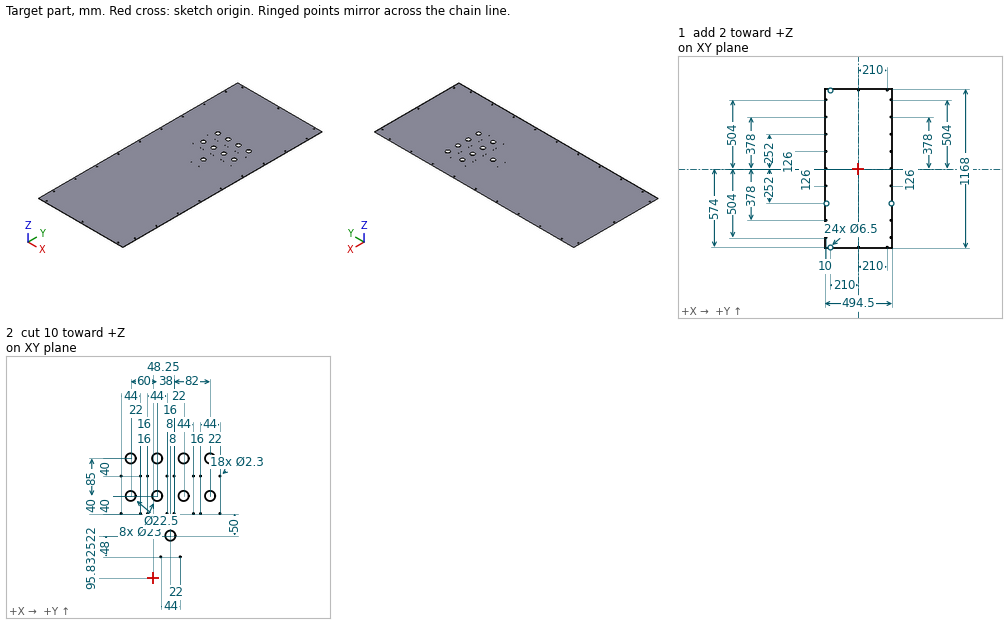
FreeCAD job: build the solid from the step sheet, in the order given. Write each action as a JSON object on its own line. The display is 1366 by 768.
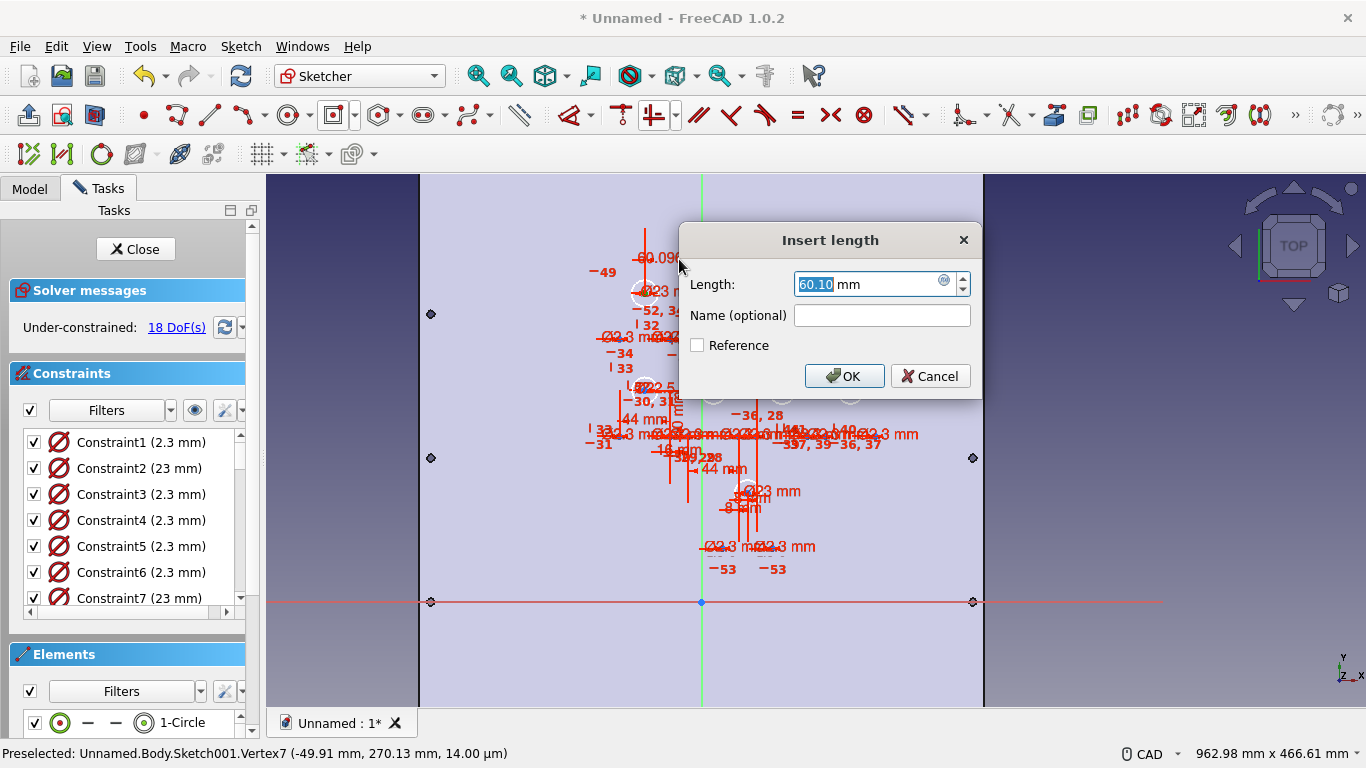
{"action": "type", "text": "60"}
{"action": "key", "text": "Return"}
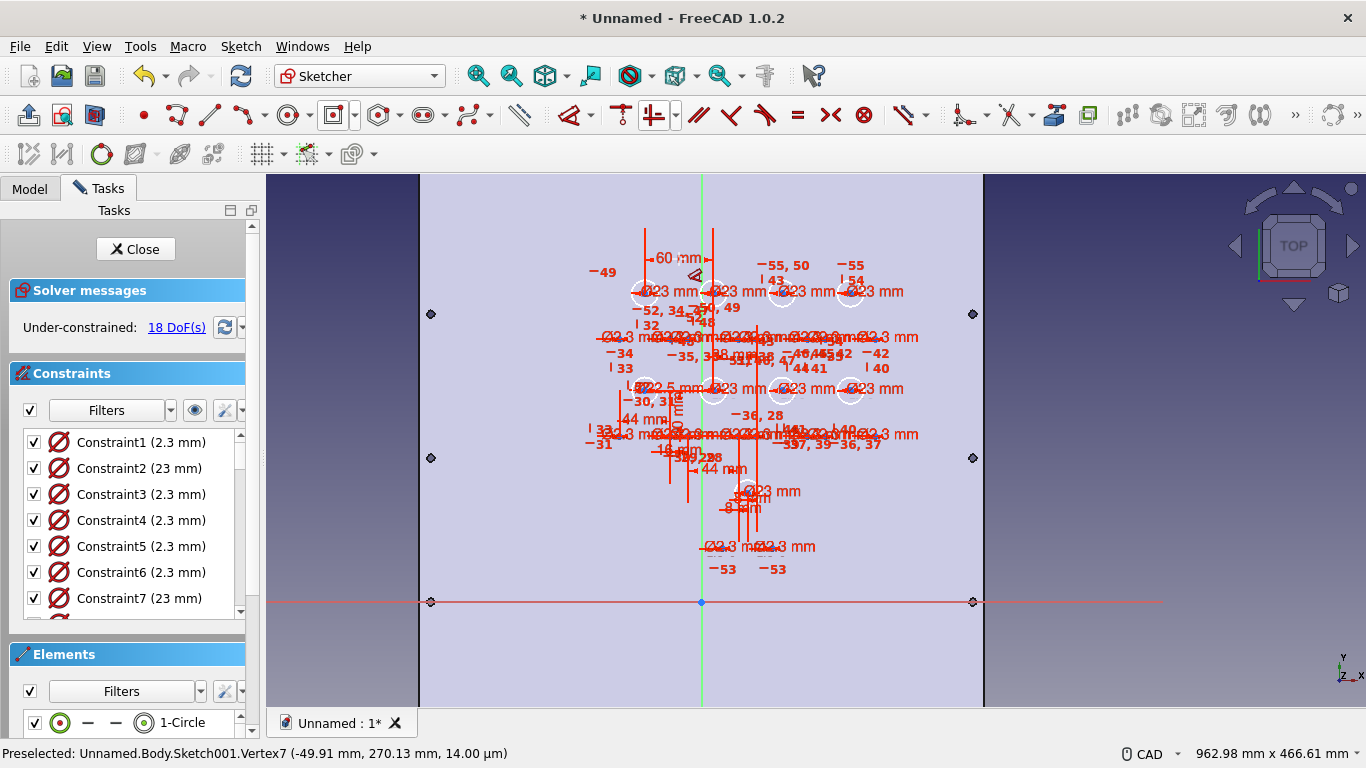
{"action": "left_click", "coordinate": [713, 391]}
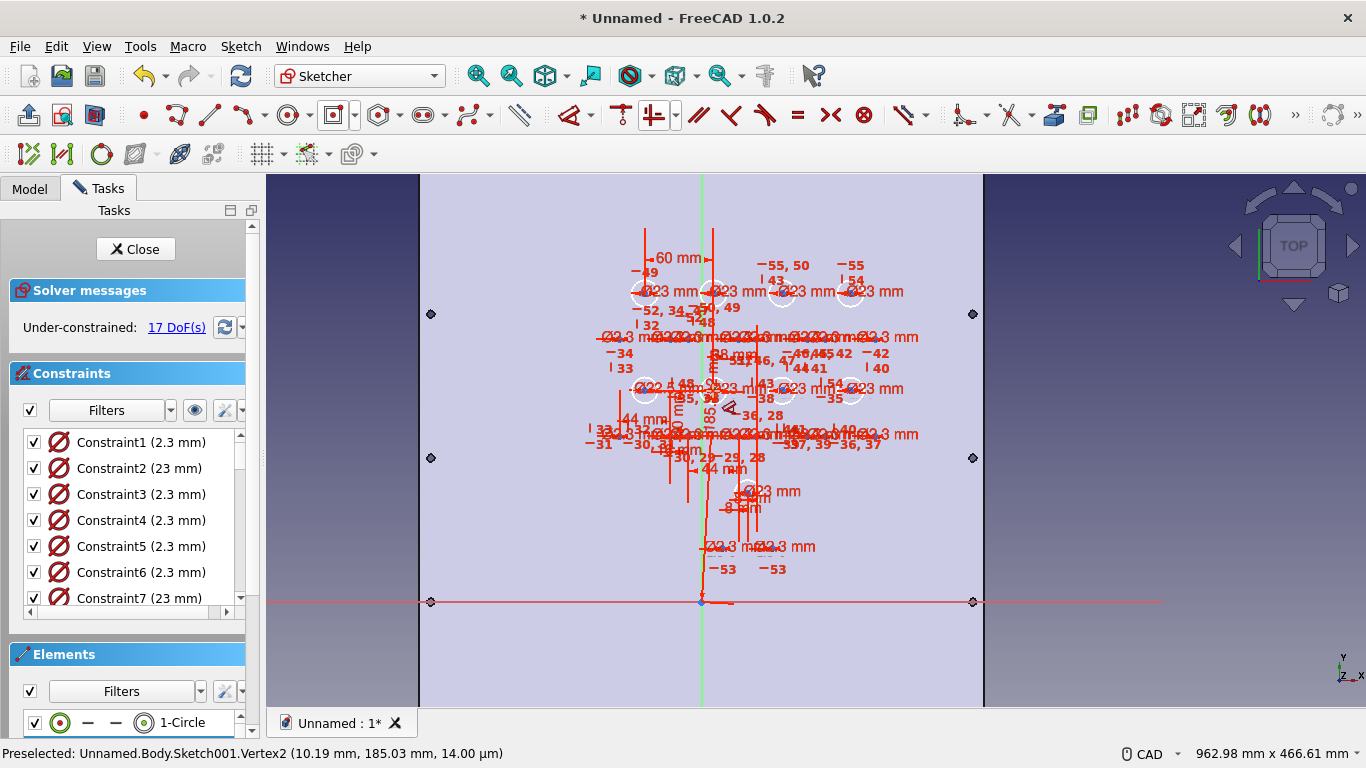
{"action": "left_click", "coordinate": [645, 293]}
{"action": "left_click", "coordinate": [611, 320]}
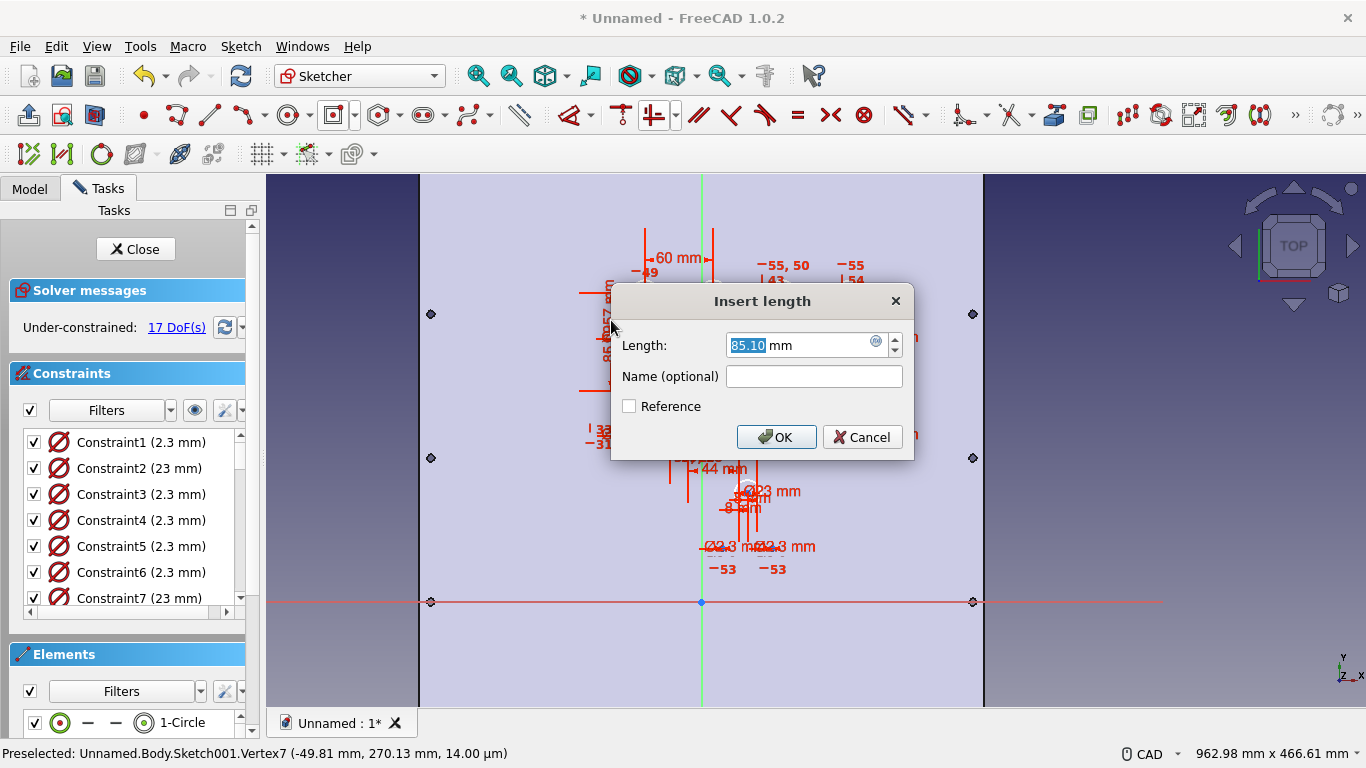
{"action": "type", "text": "85"}
{"action": "key", "text": "Return"}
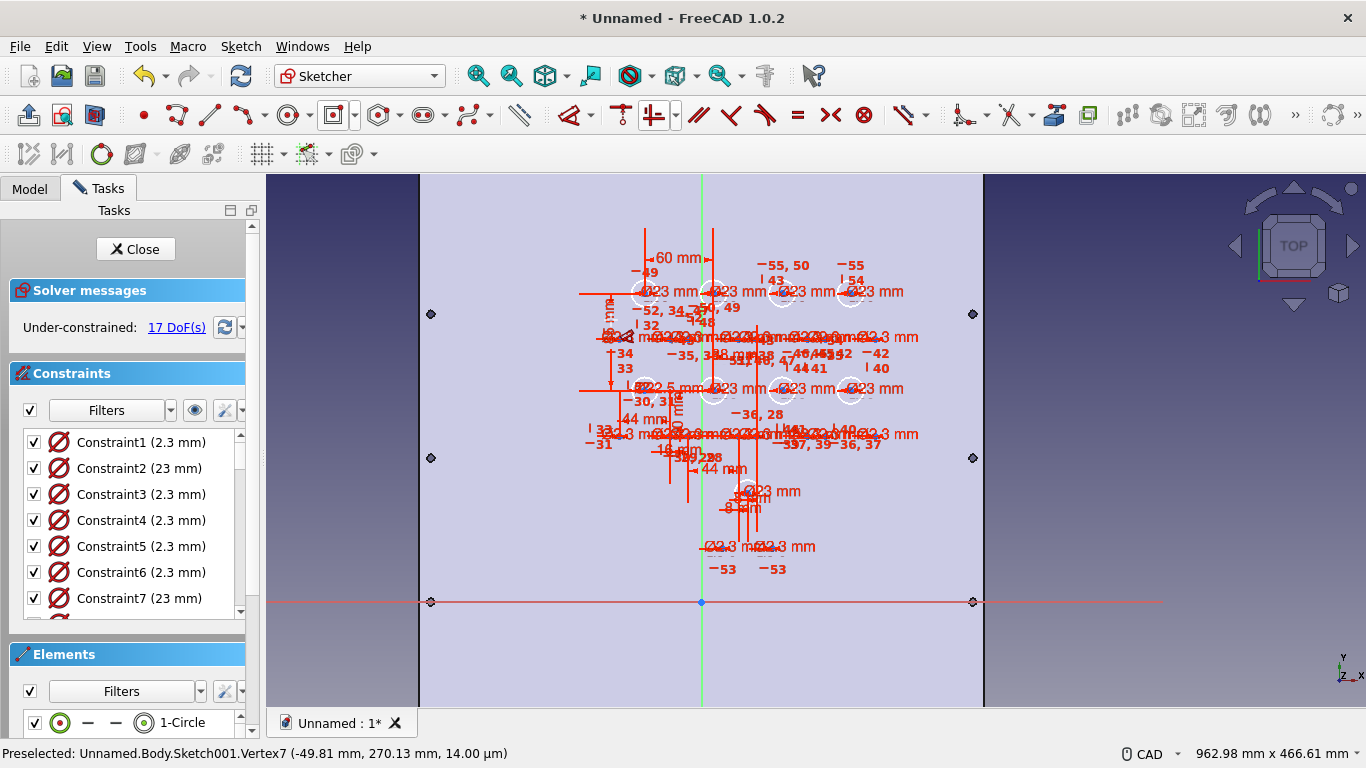
{"action": "left_click", "coordinate": [645, 294]}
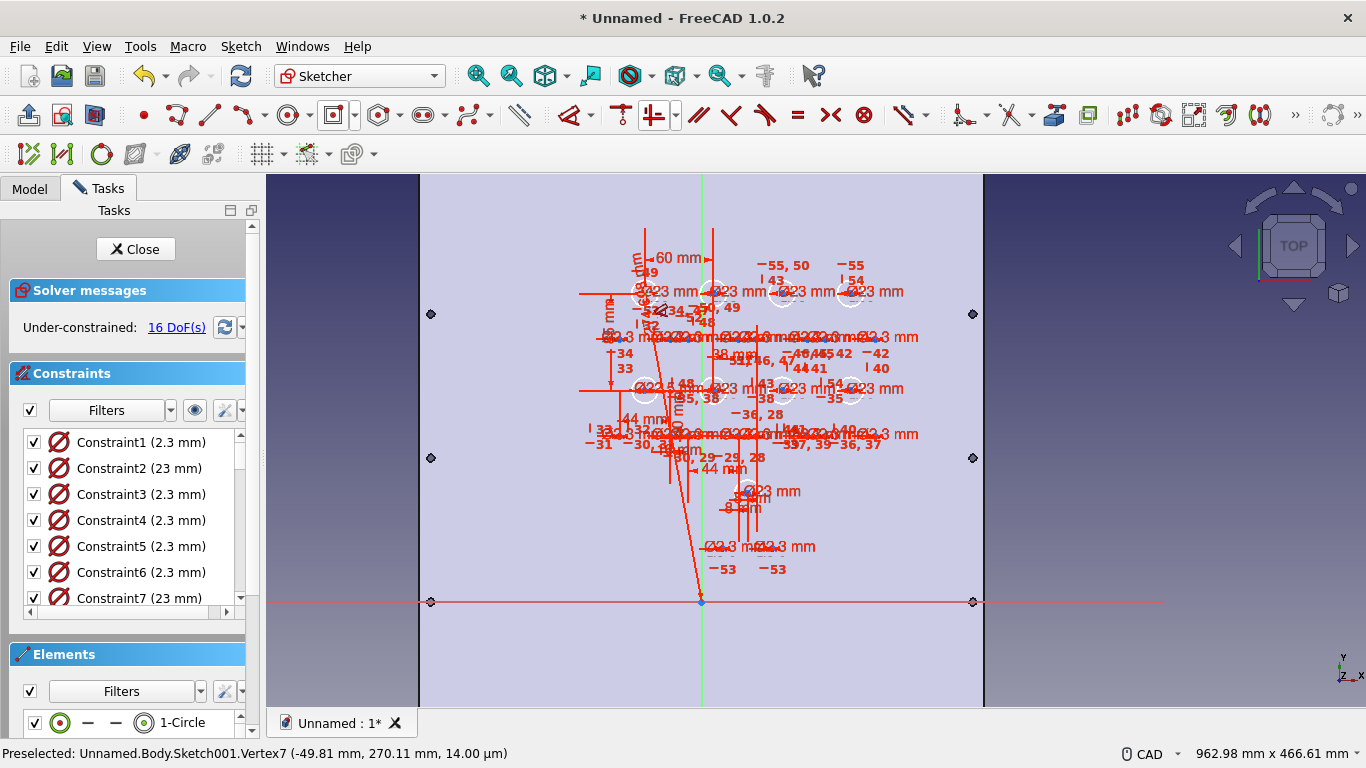
{"action": "left_click", "coordinate": [670, 339]}
{"action": "left_click", "coordinate": [728, 316]}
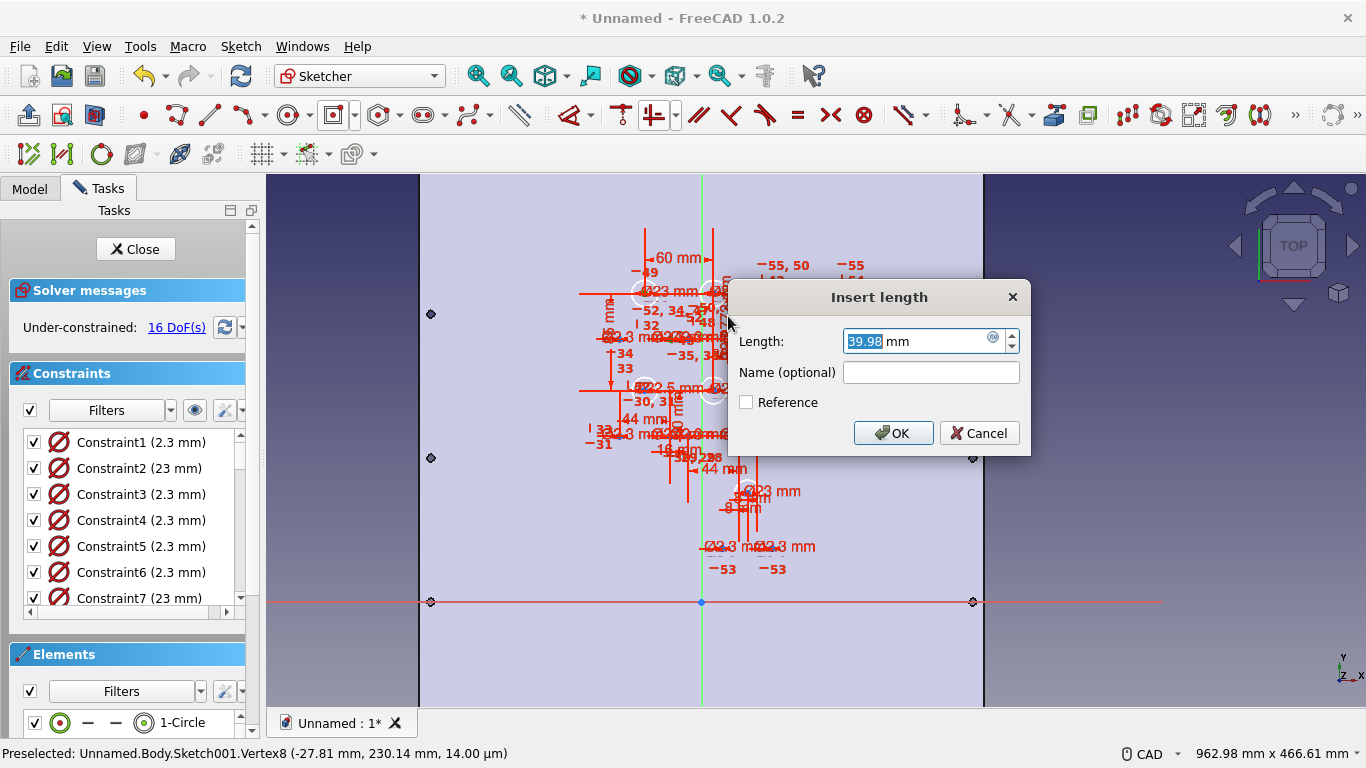
{"action": "type", "text": "40"}
{"action": "key", "text": "Return"}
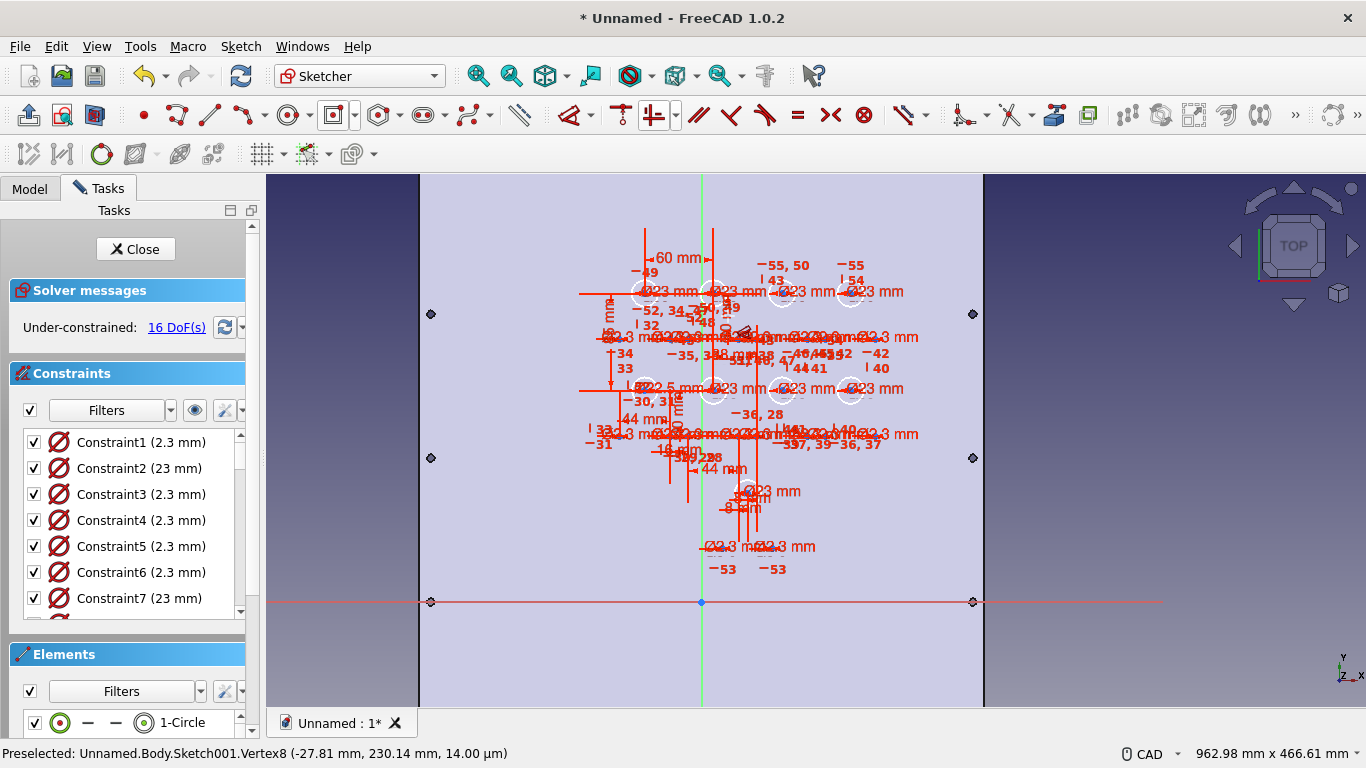
{"action": "left_click", "coordinate": [757, 436]}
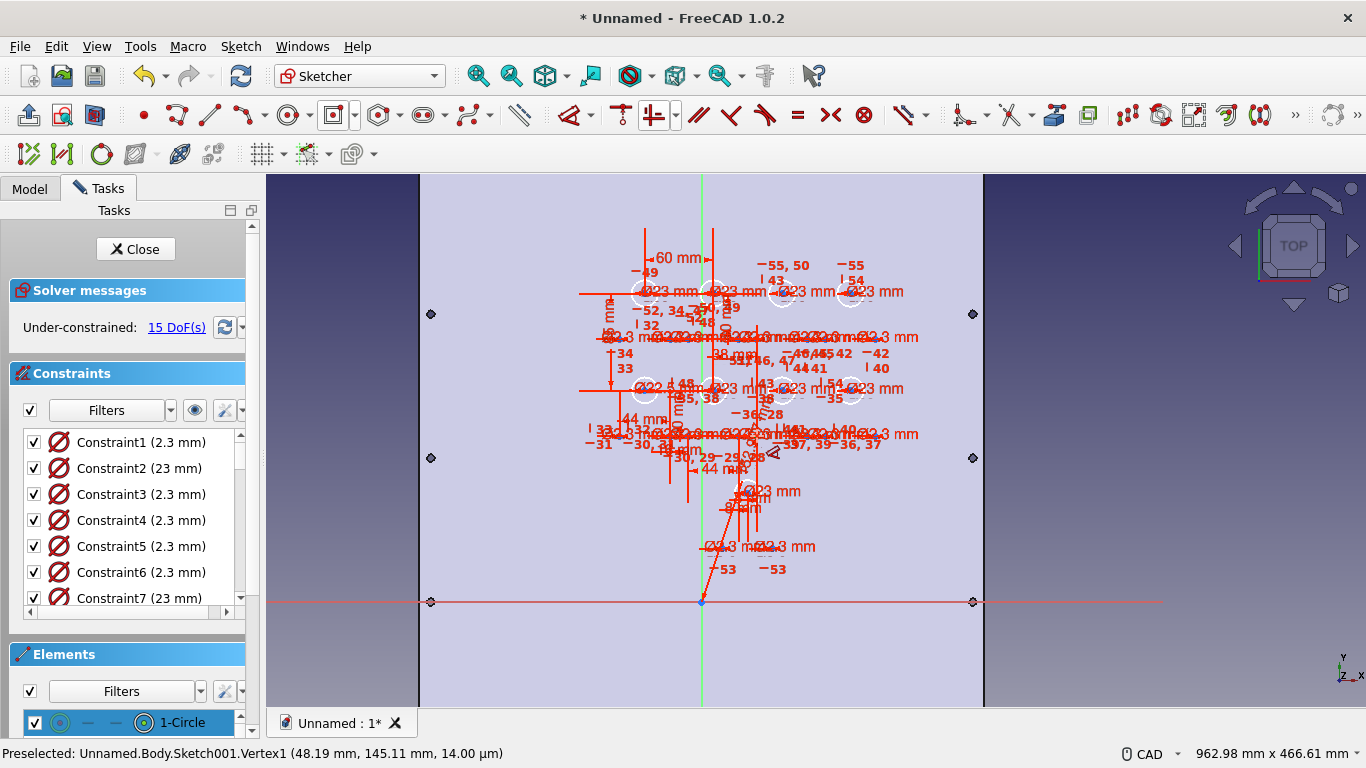
{"action": "left_click", "coordinate": [851, 391]}
{"action": "left_click", "coordinate": [825, 357]}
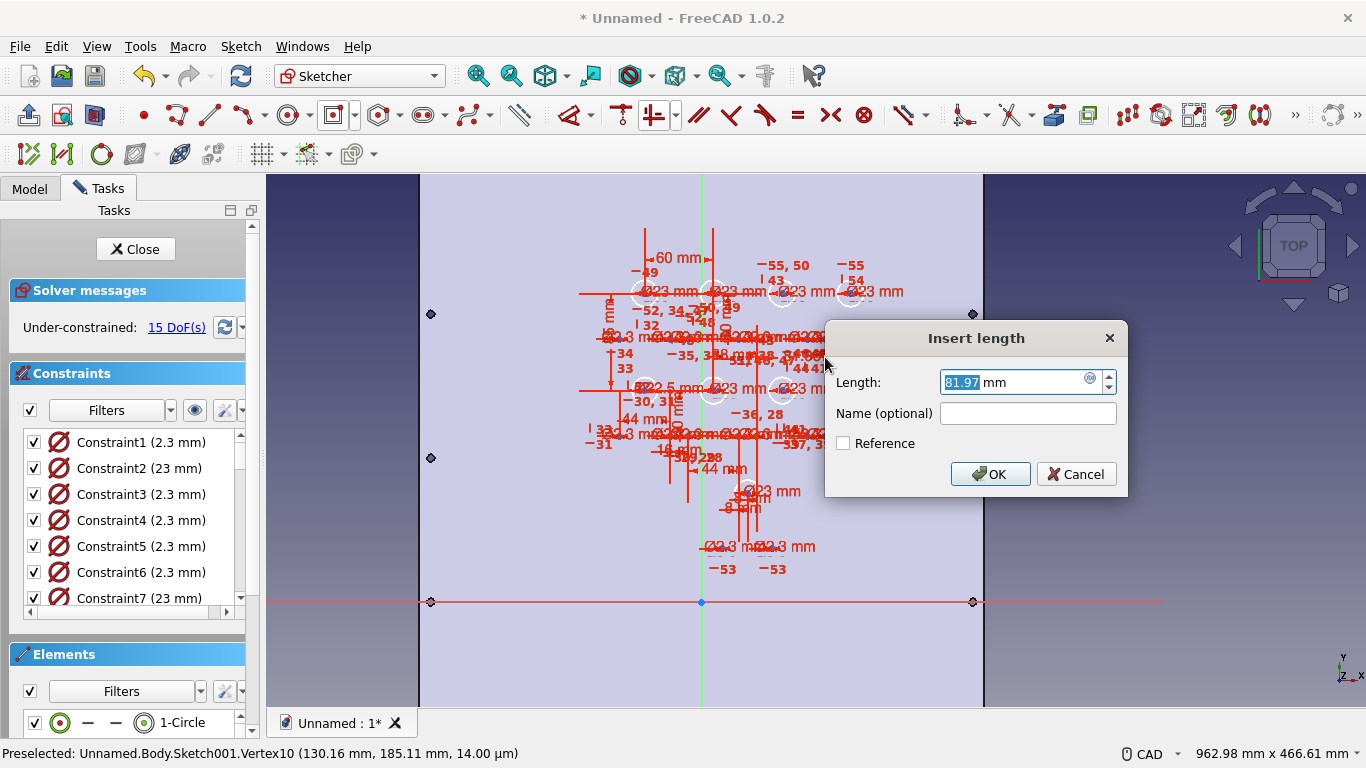
{"action": "type", "text": "82"}
{"action": "key", "text": "Return"}